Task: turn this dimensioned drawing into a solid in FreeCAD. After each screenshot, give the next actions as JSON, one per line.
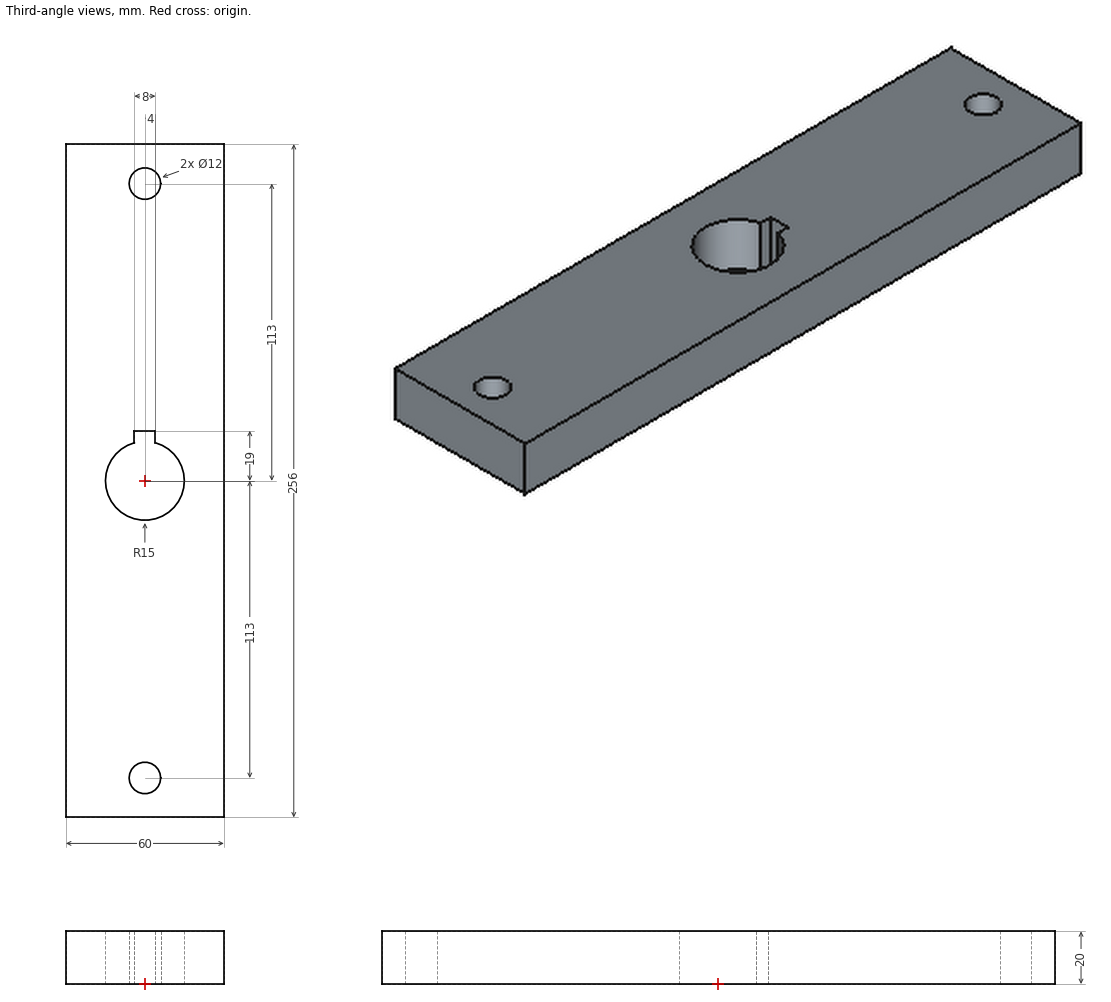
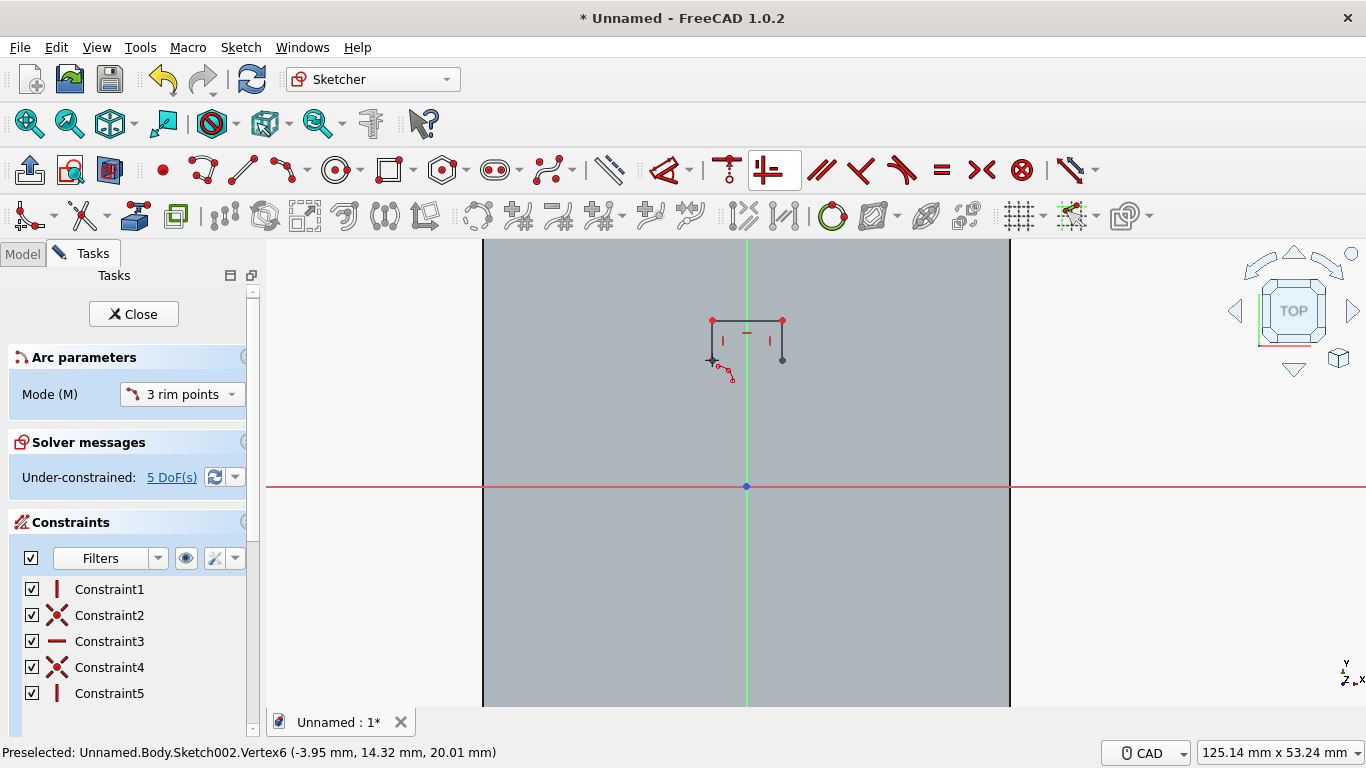
{"action": "left_click", "coordinate": [712, 361]}
{"action": "left_click", "coordinate": [782, 361]}
{"action": "left_click", "coordinate": [675, 598]}
{"action": "key", "text": "Escape"}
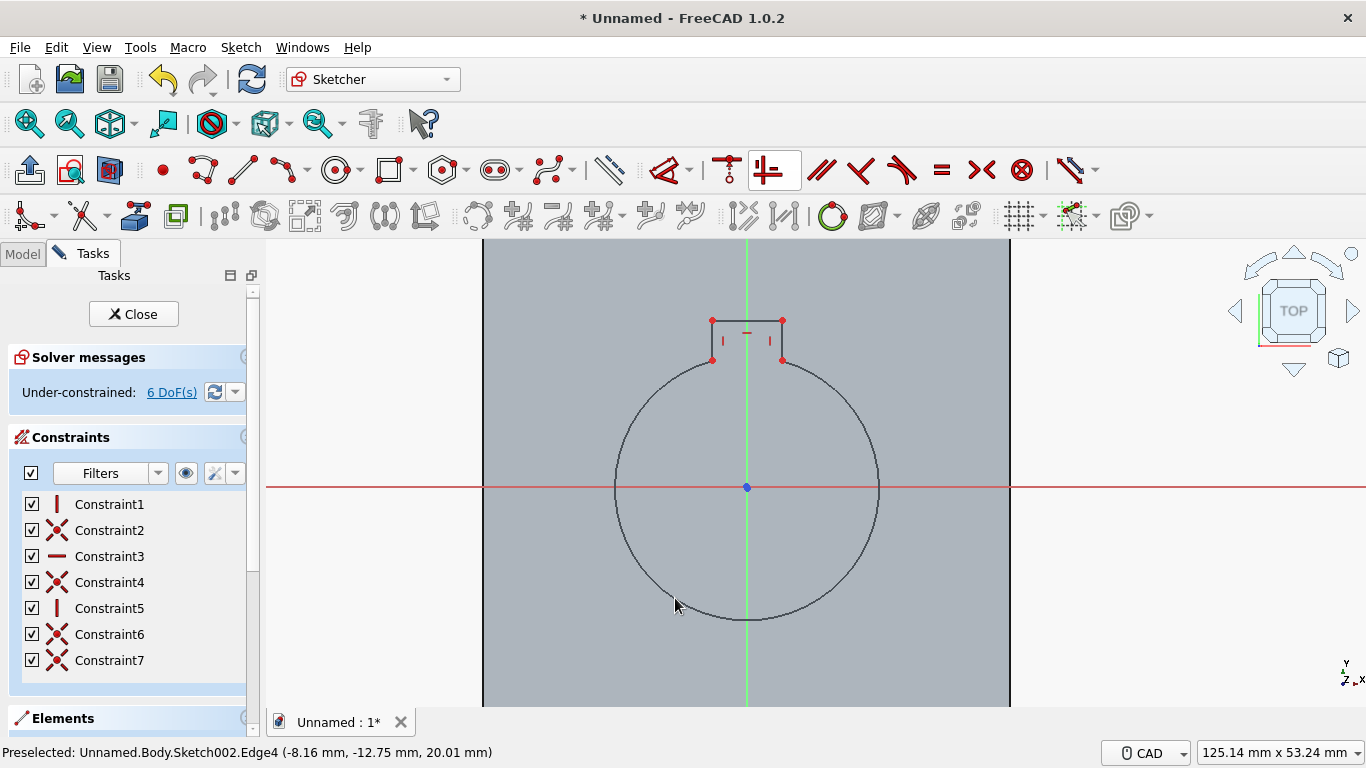
{"action": "left_click_drag", "start_coordinate": [737, 477], "coordinate": [757, 498]}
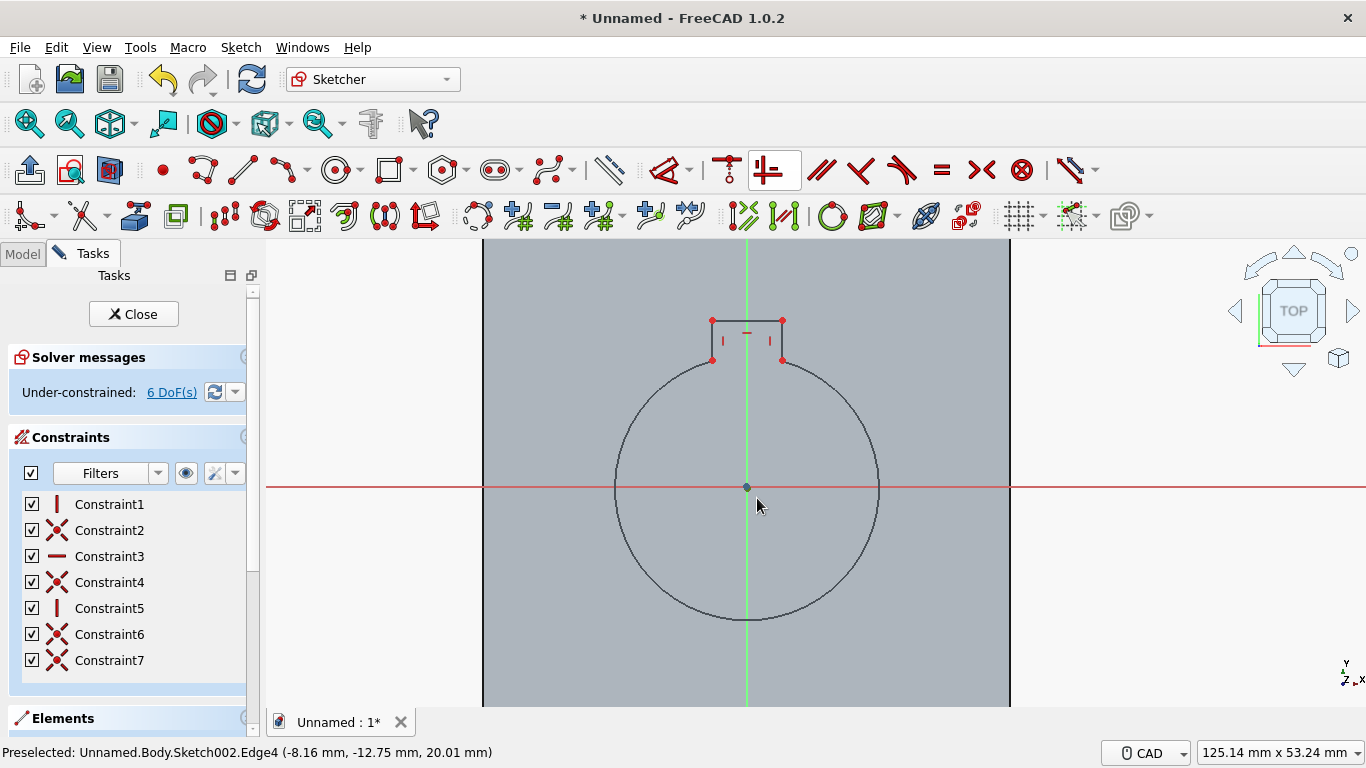
{"action": "left_click", "coordinate": [728, 170]}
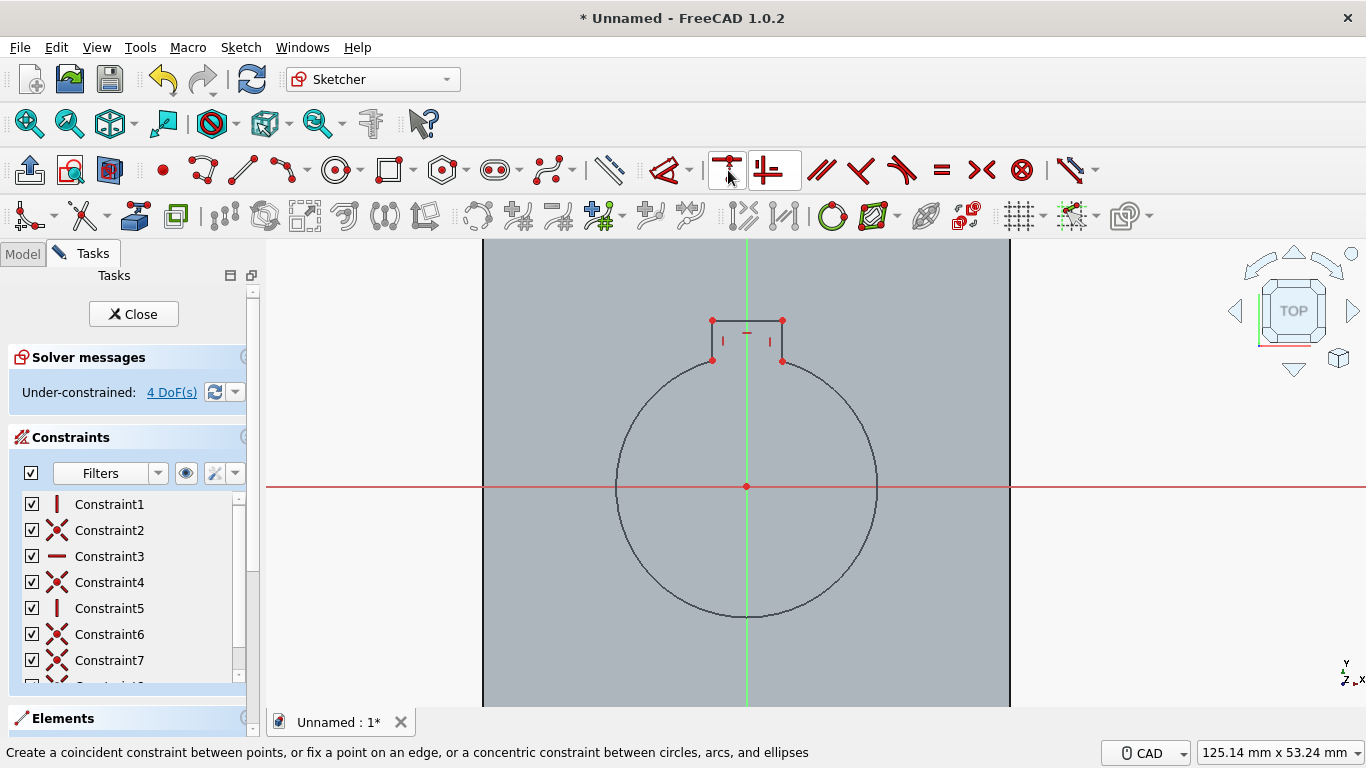
{"action": "key", "text": "d"}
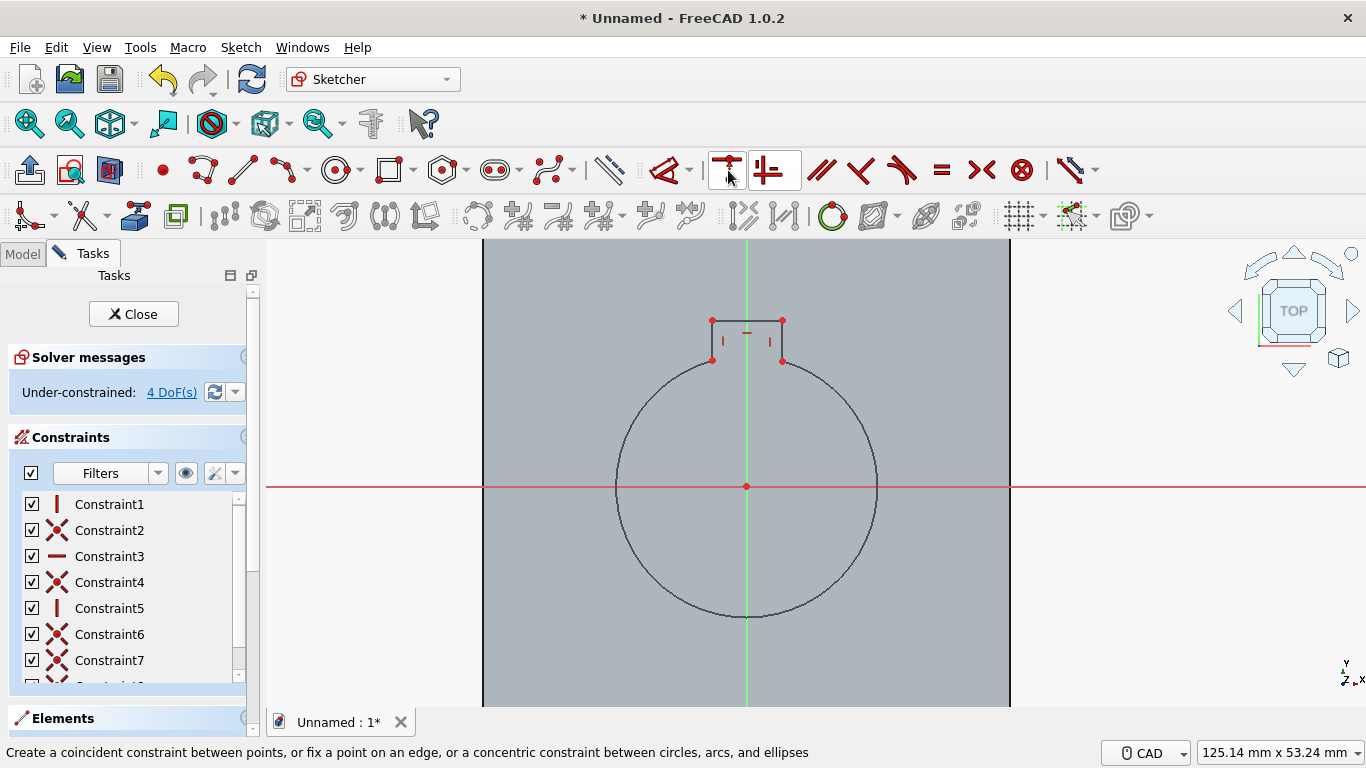
{"action": "left_click", "coordinate": [627, 540]}
{"action": "left_click", "coordinate": [598, 553]}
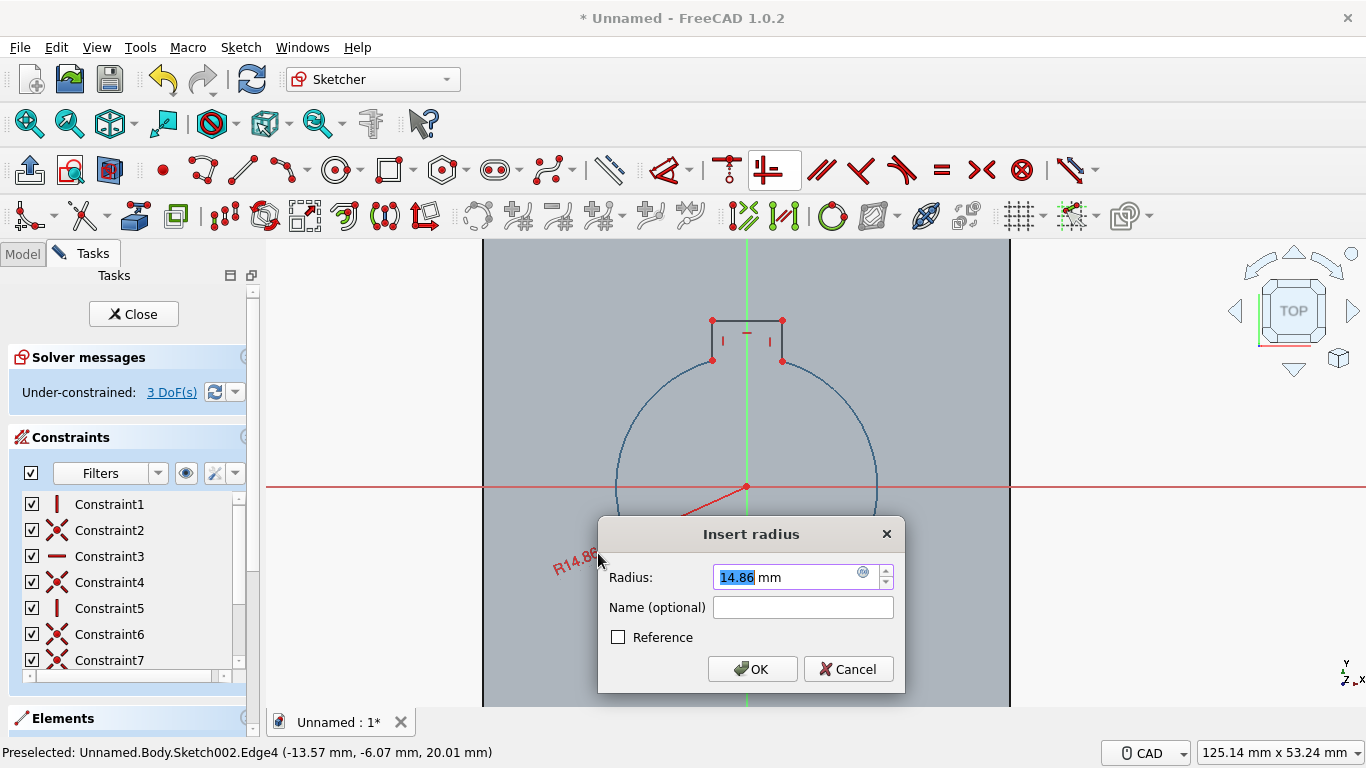
{"action": "type", "text": "15"}
{"action": "key", "text": "Return"}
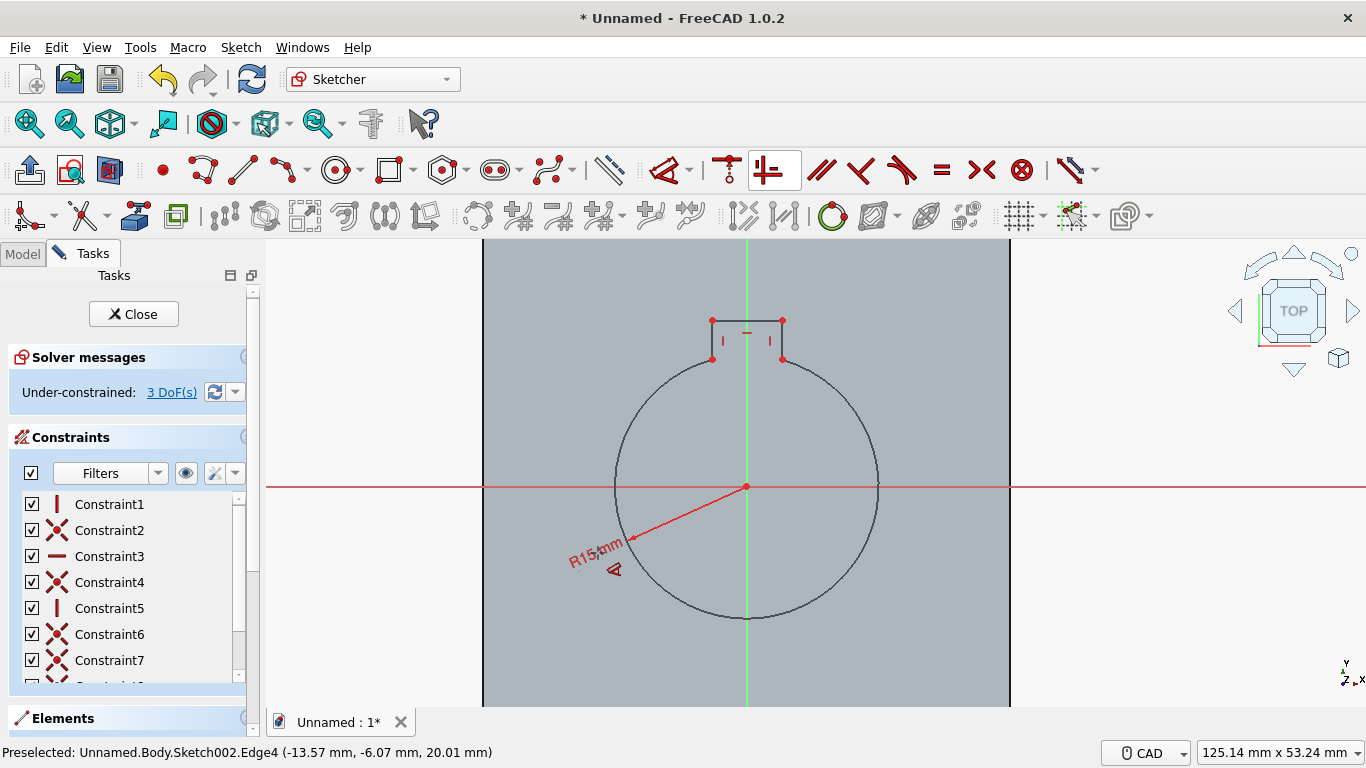
{"action": "left_click", "coordinate": [761, 321]}
{"action": "left_click", "coordinate": [731, 287]}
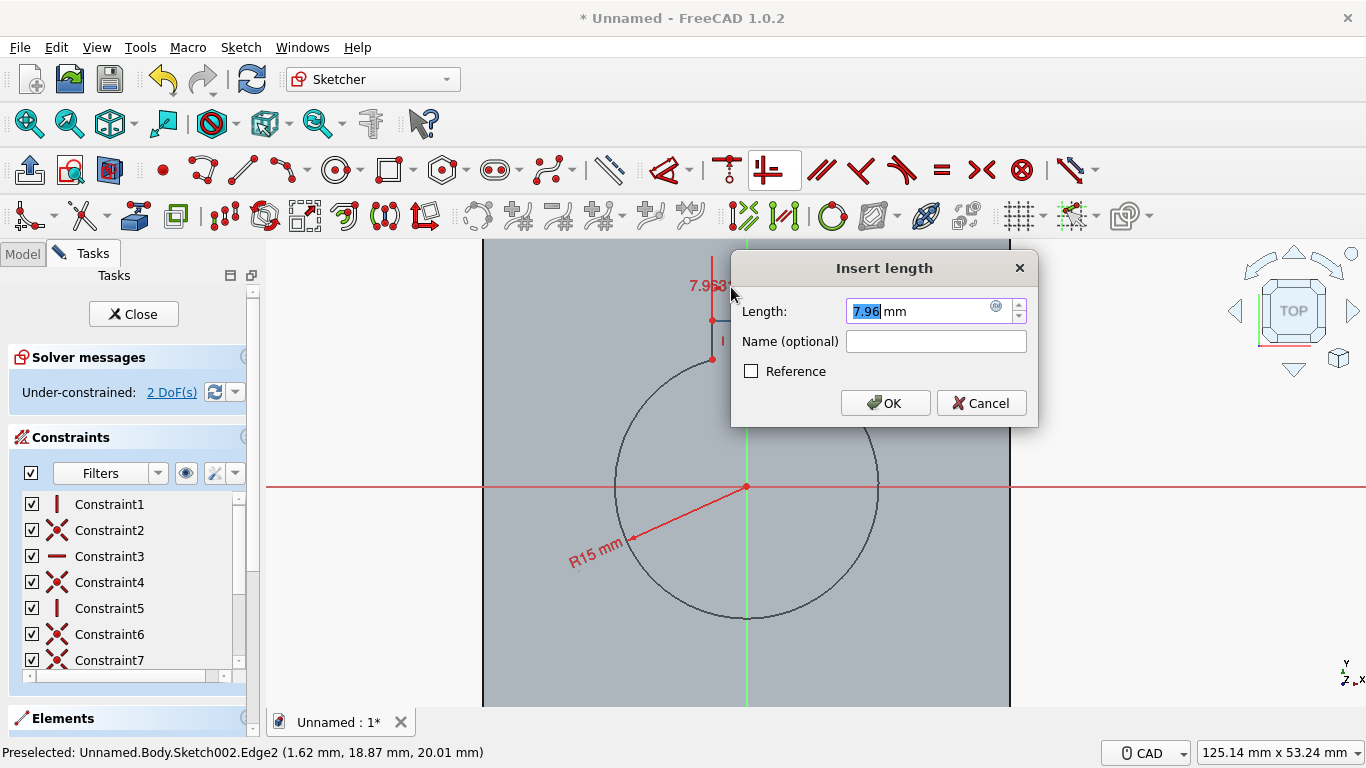
{"action": "type", "text": "8"}
{"action": "key", "text": "Return"}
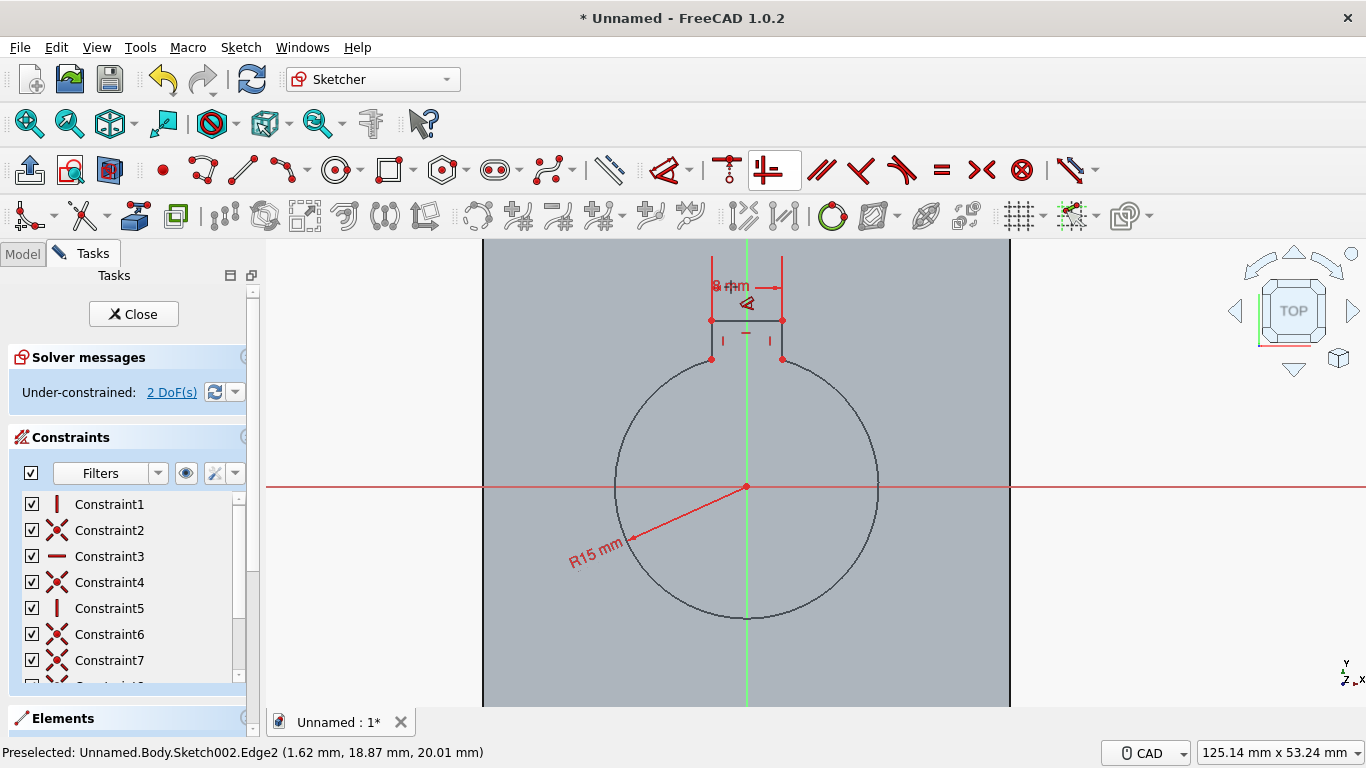
{"action": "left_click", "coordinate": [782, 360]}
{"action": "left_click", "coordinate": [764, 521]}